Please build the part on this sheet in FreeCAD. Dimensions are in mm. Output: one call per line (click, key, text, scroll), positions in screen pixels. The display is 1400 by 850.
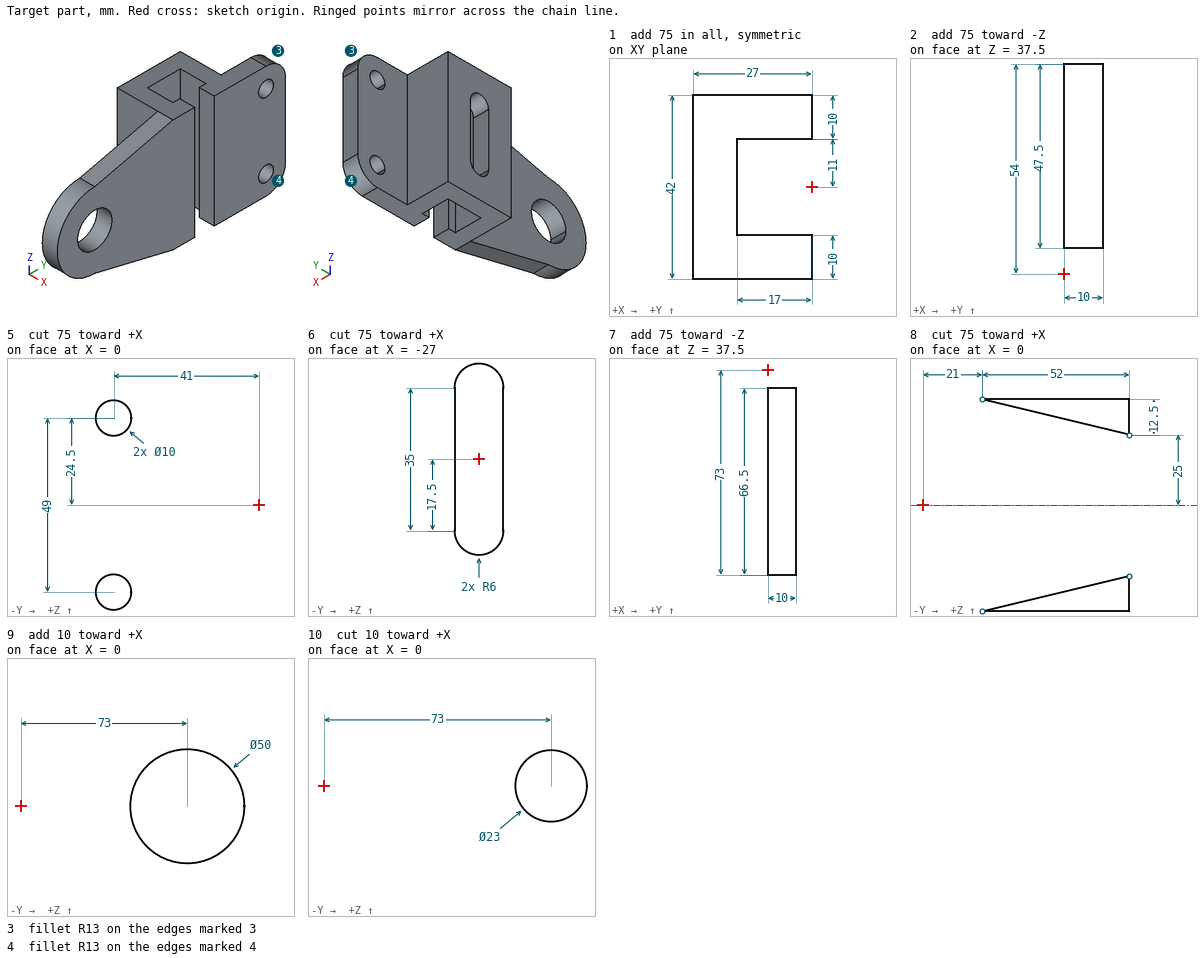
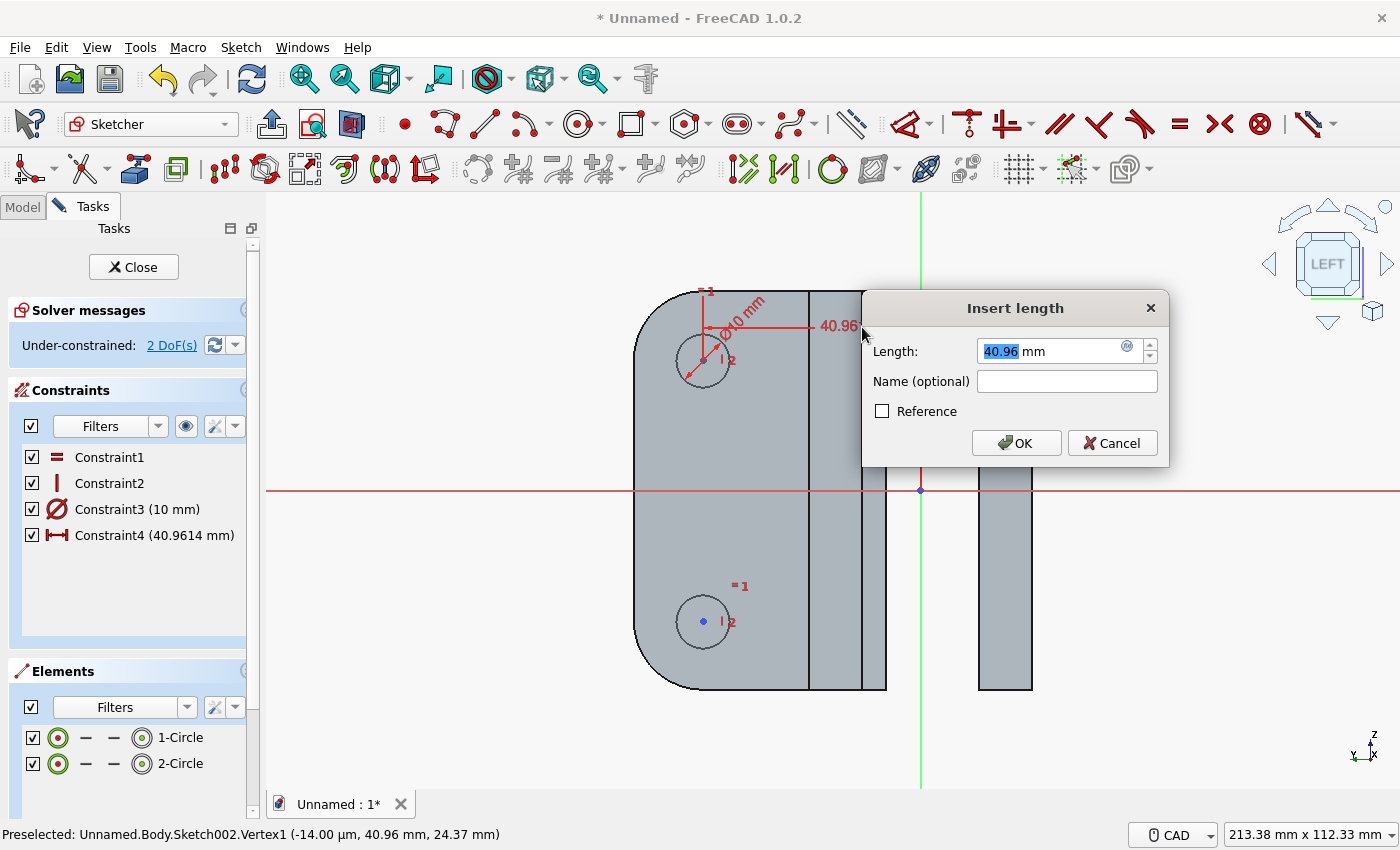
text(41)
key(Return)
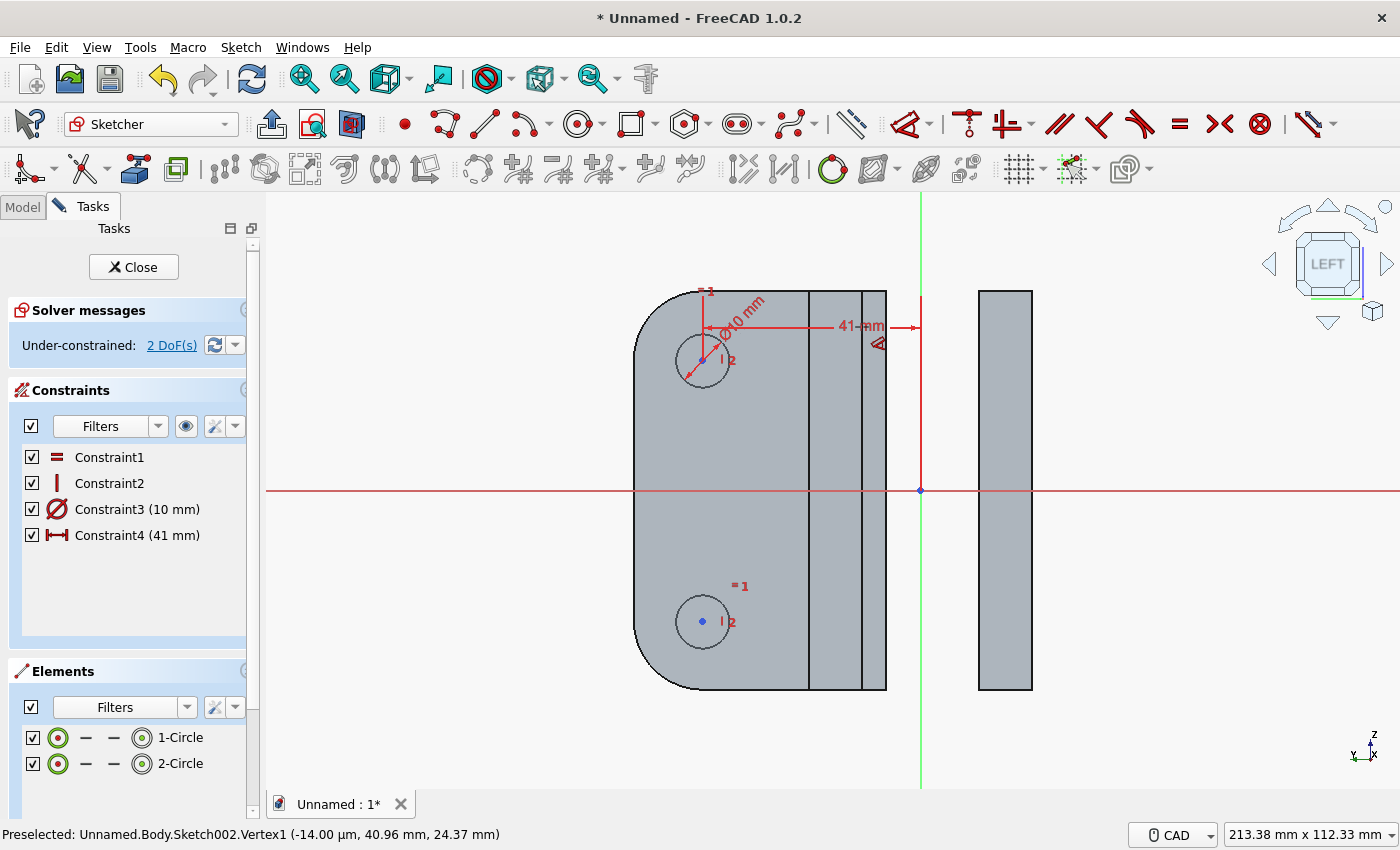
click(703, 361)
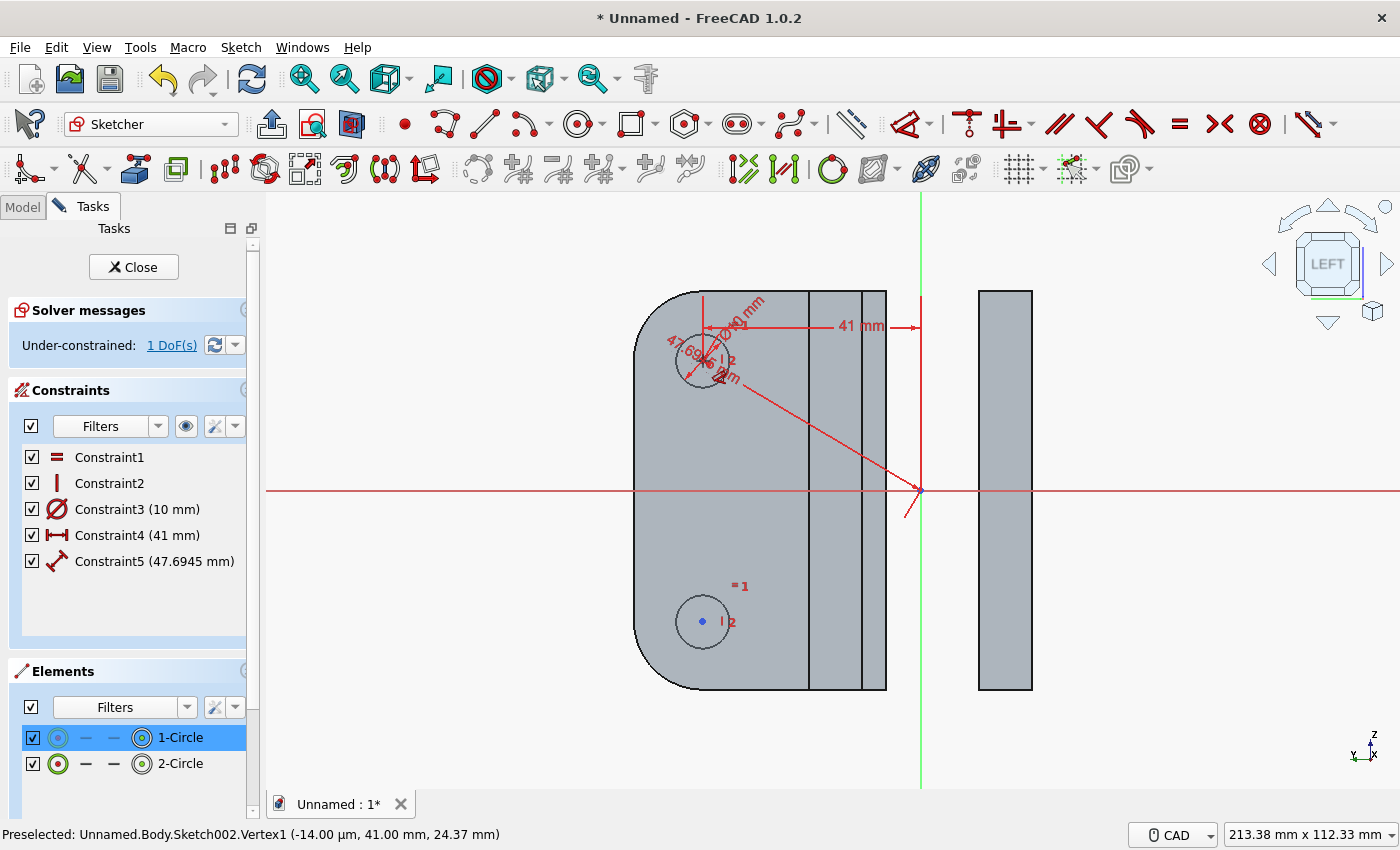
click(703, 622)
click(669, 431)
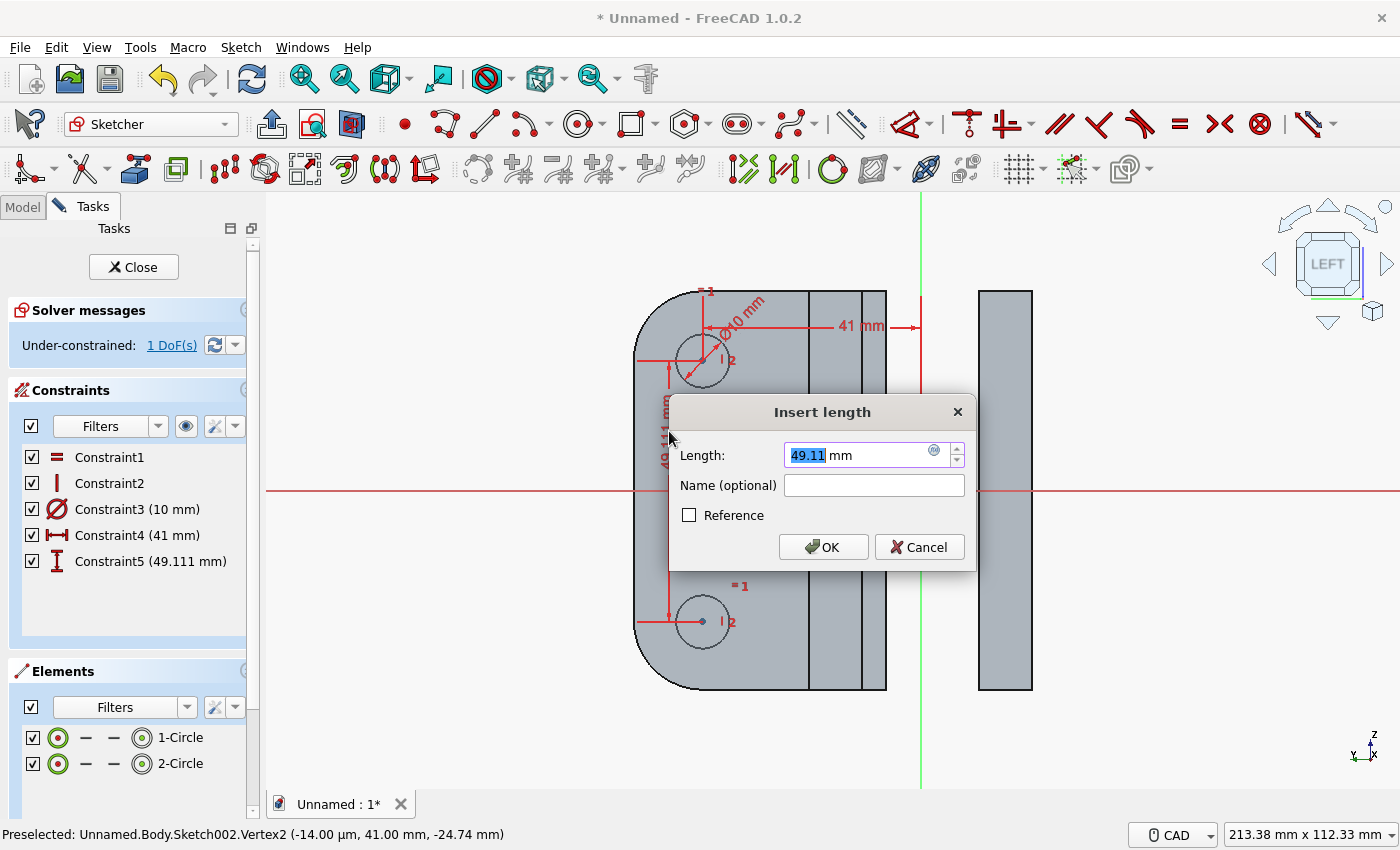
text(49)
key(Return)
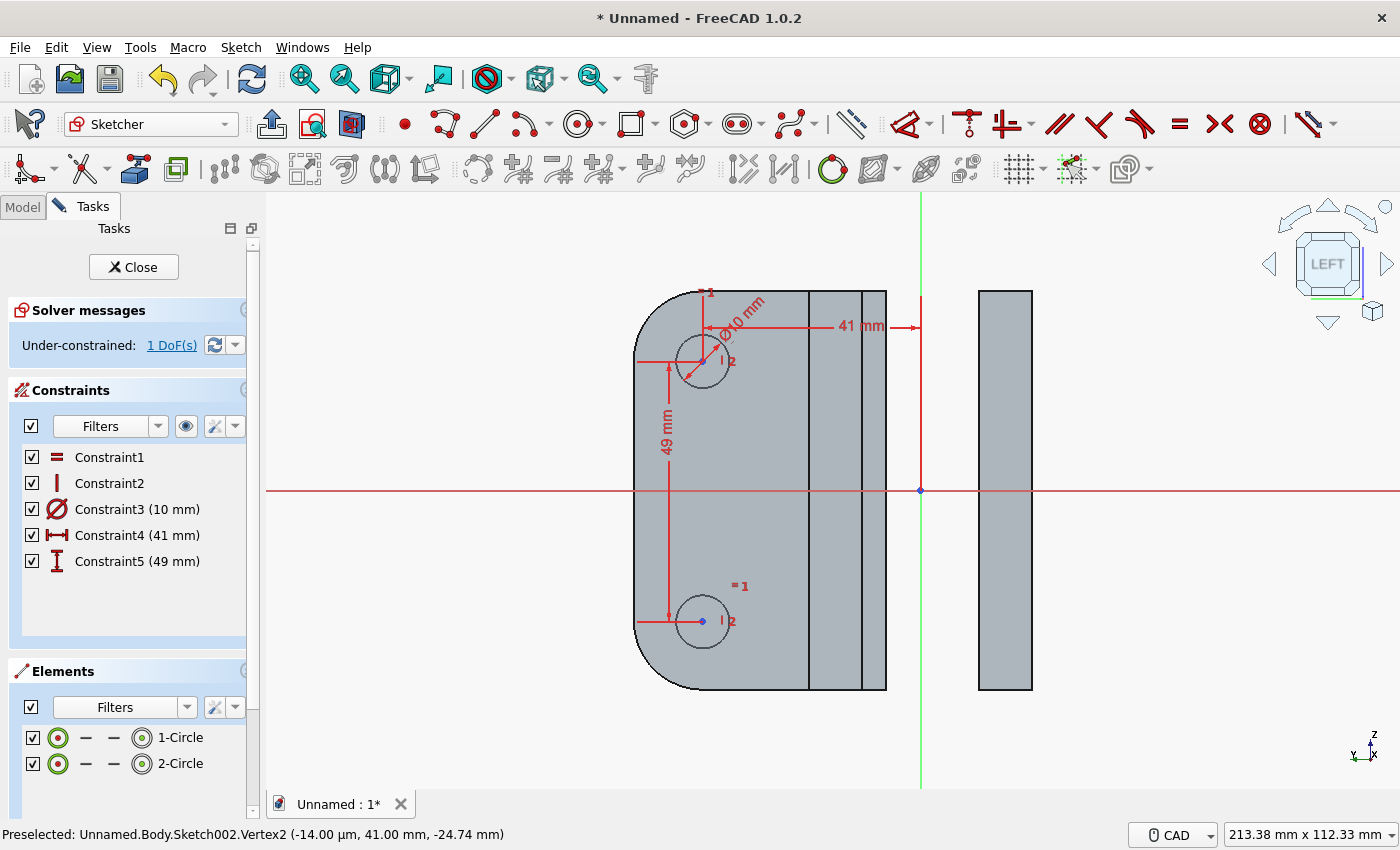
click(703, 362)
click(955, 426)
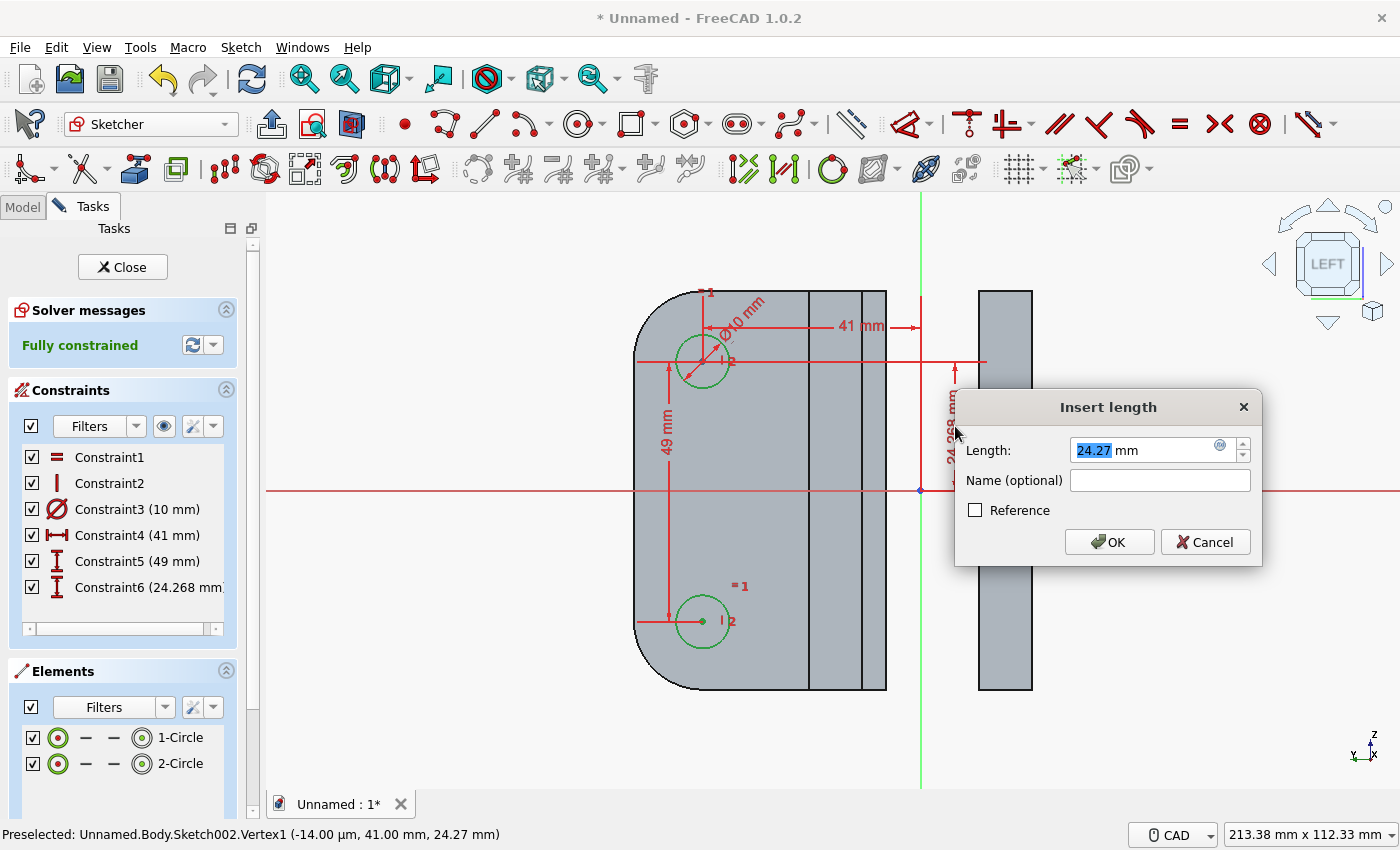
text(24.5)
key(Return)
key(Escape)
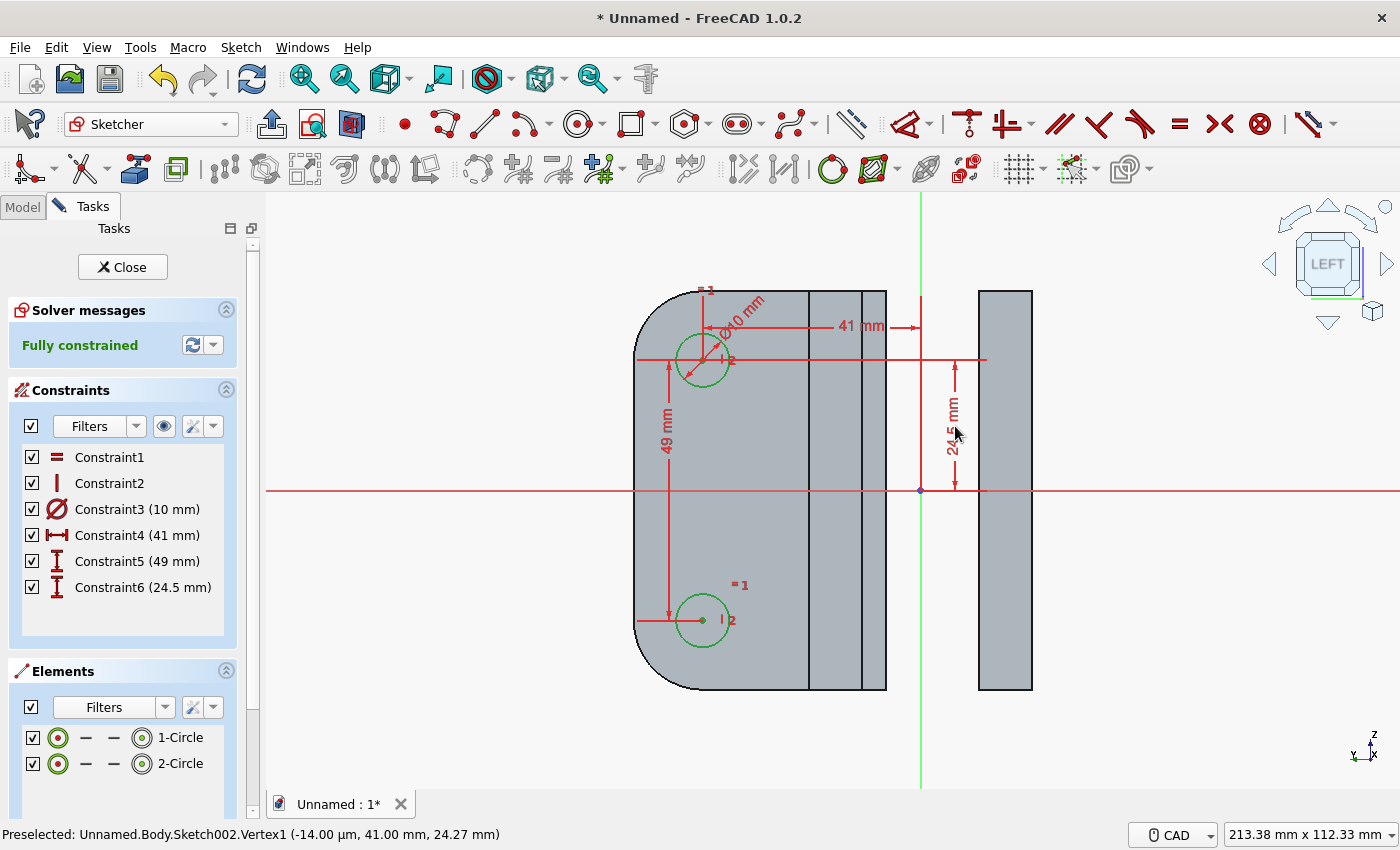
click(123, 267)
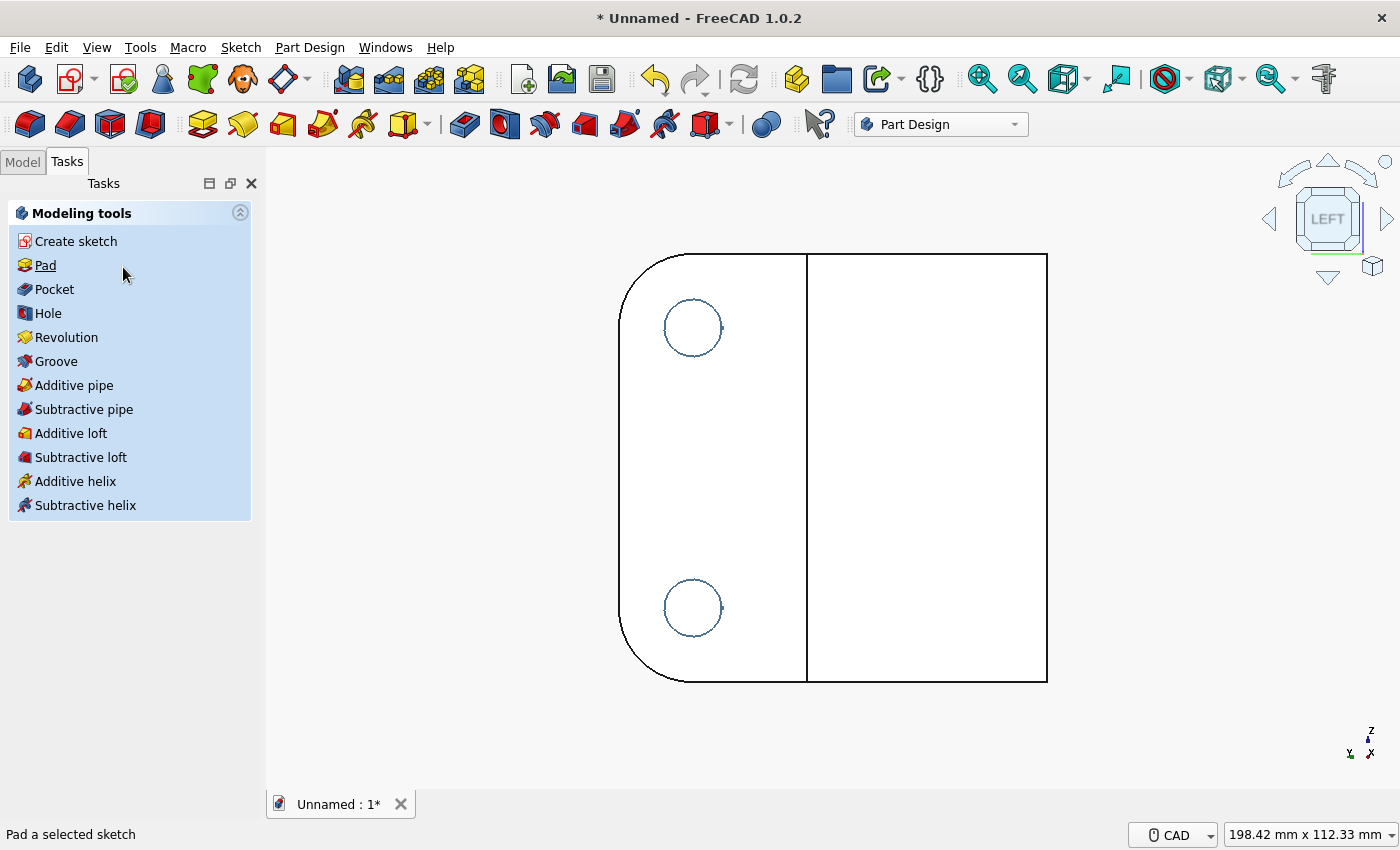
click(466, 124)